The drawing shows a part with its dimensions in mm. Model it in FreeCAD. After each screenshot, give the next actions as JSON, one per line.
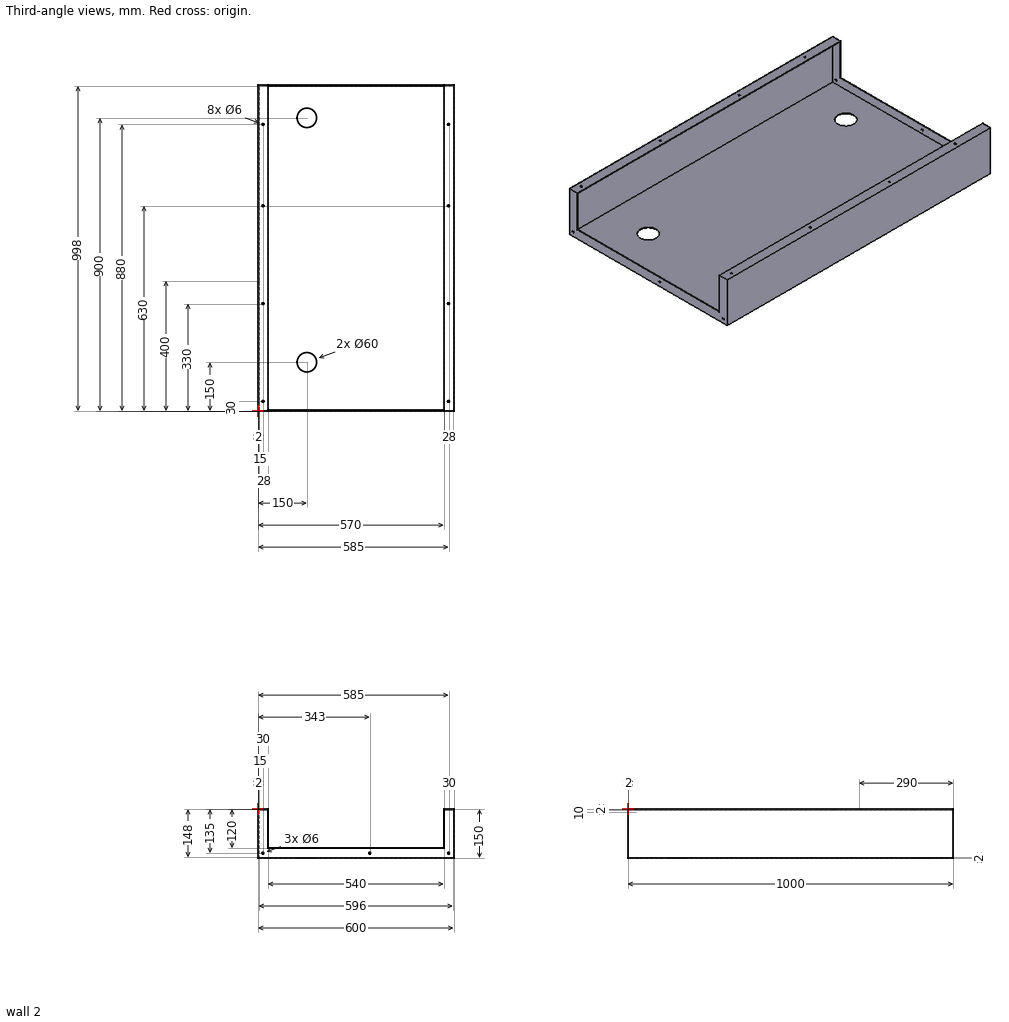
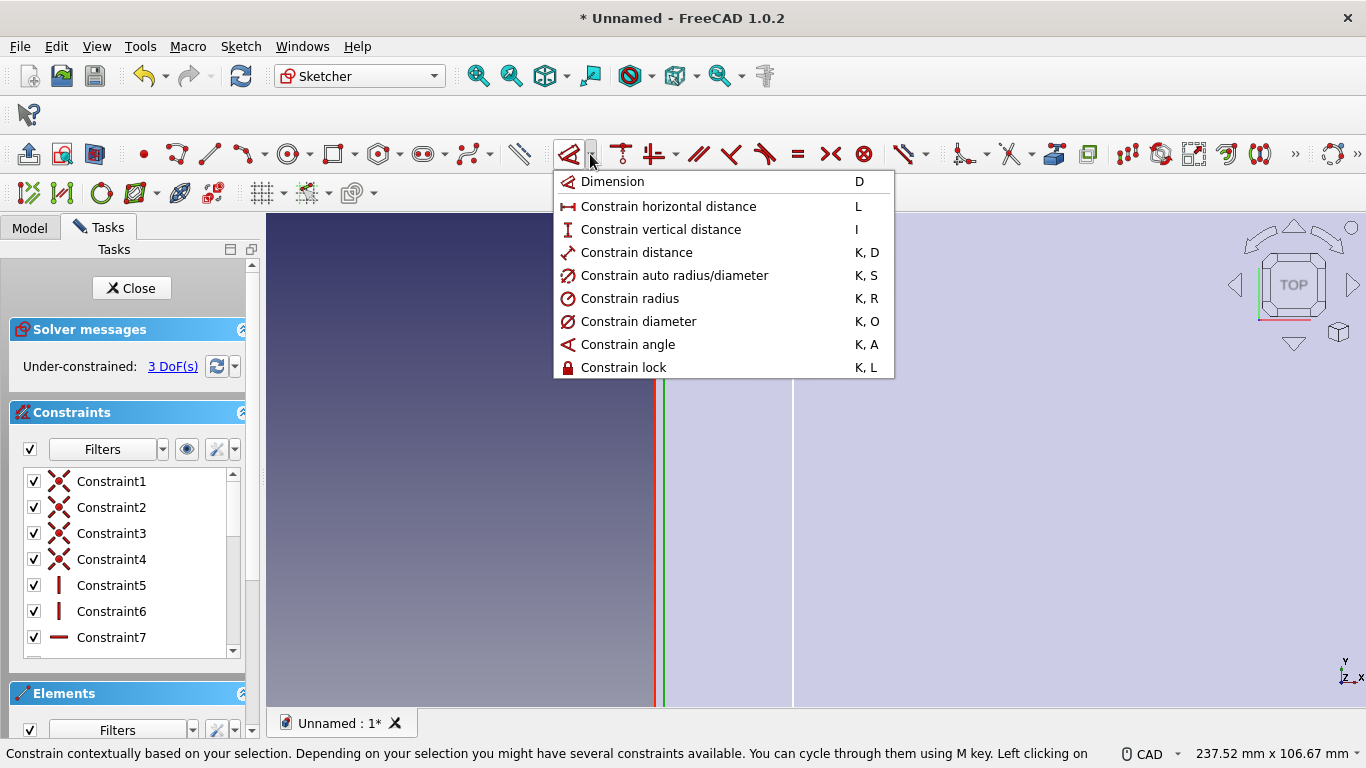
{"action": "left_click", "coordinate": [724, 230]}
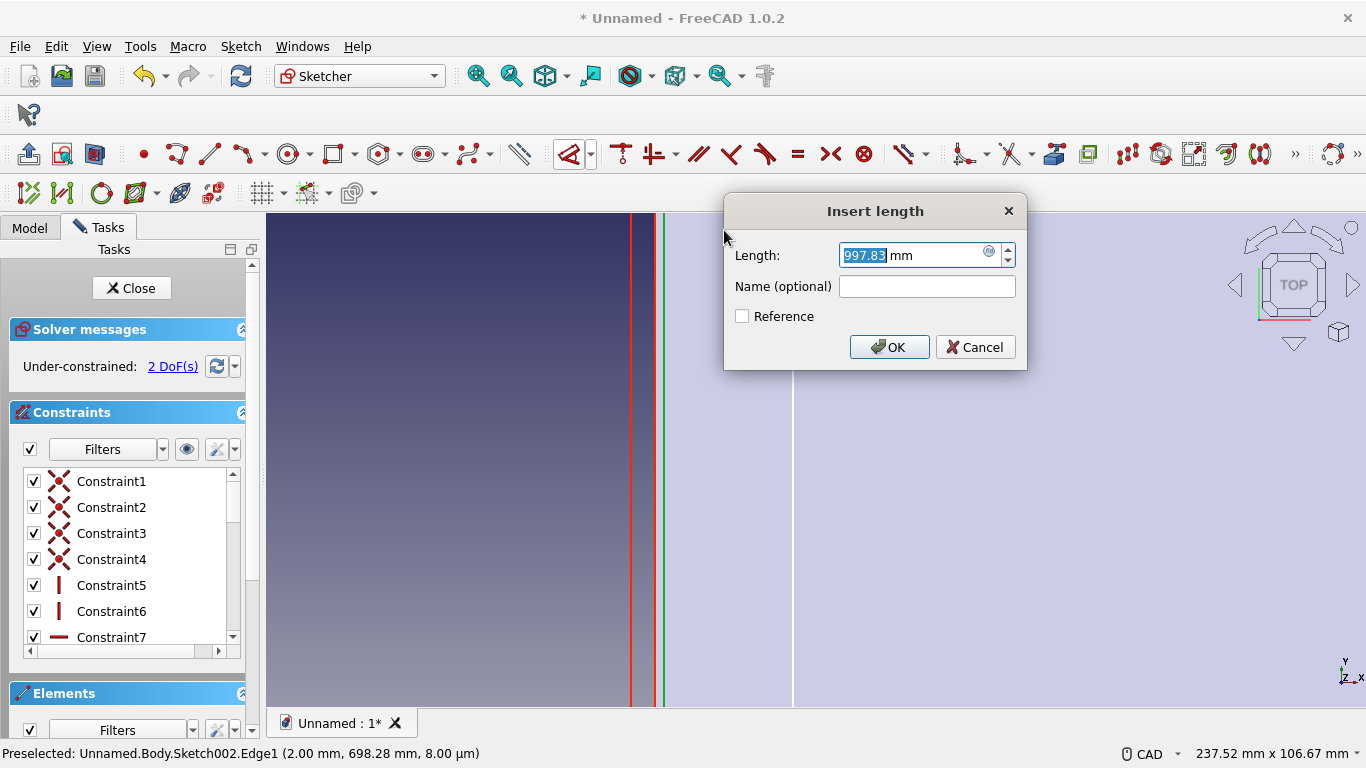
{"action": "type", "text": "998"}
{"action": "key", "text": "Return"}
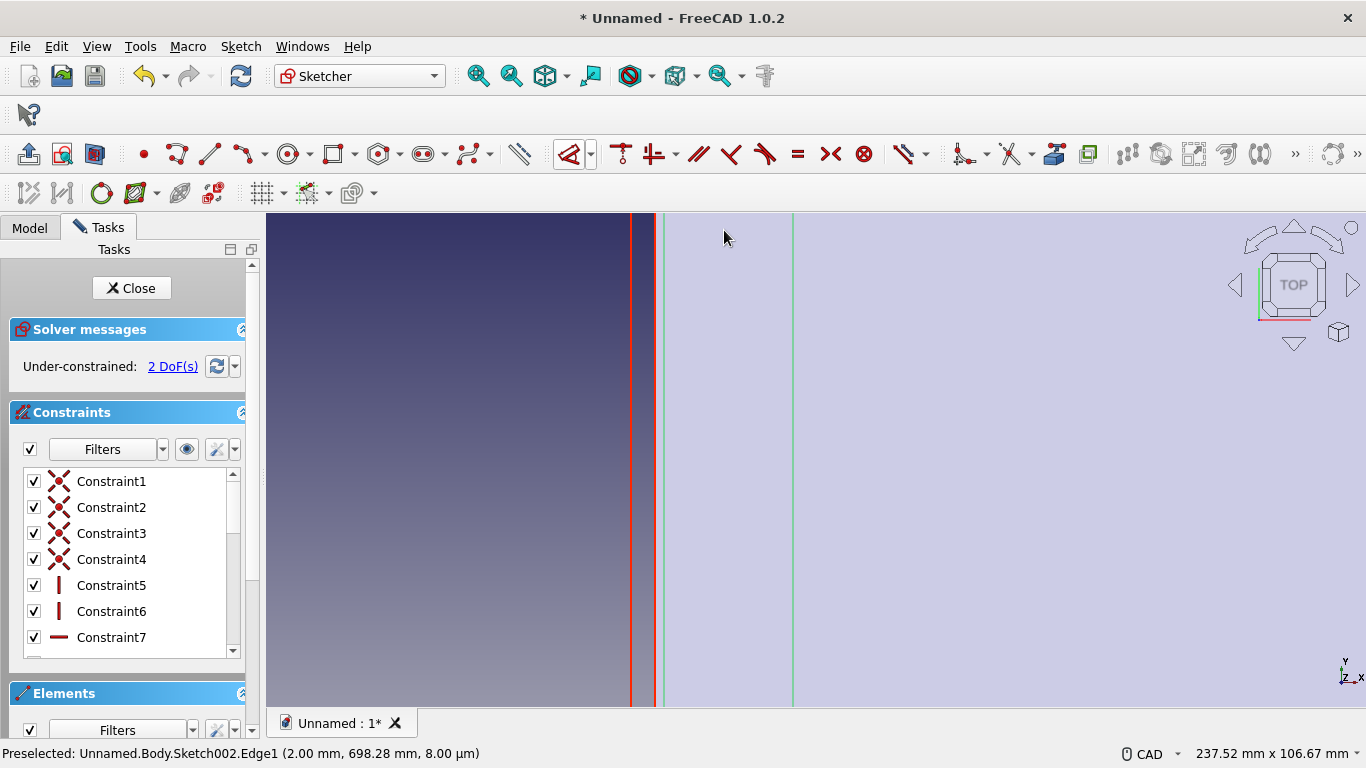
{"action": "scroll", "coordinate": [664, 405], "scroll_direction": "down", "scroll_amount": 14}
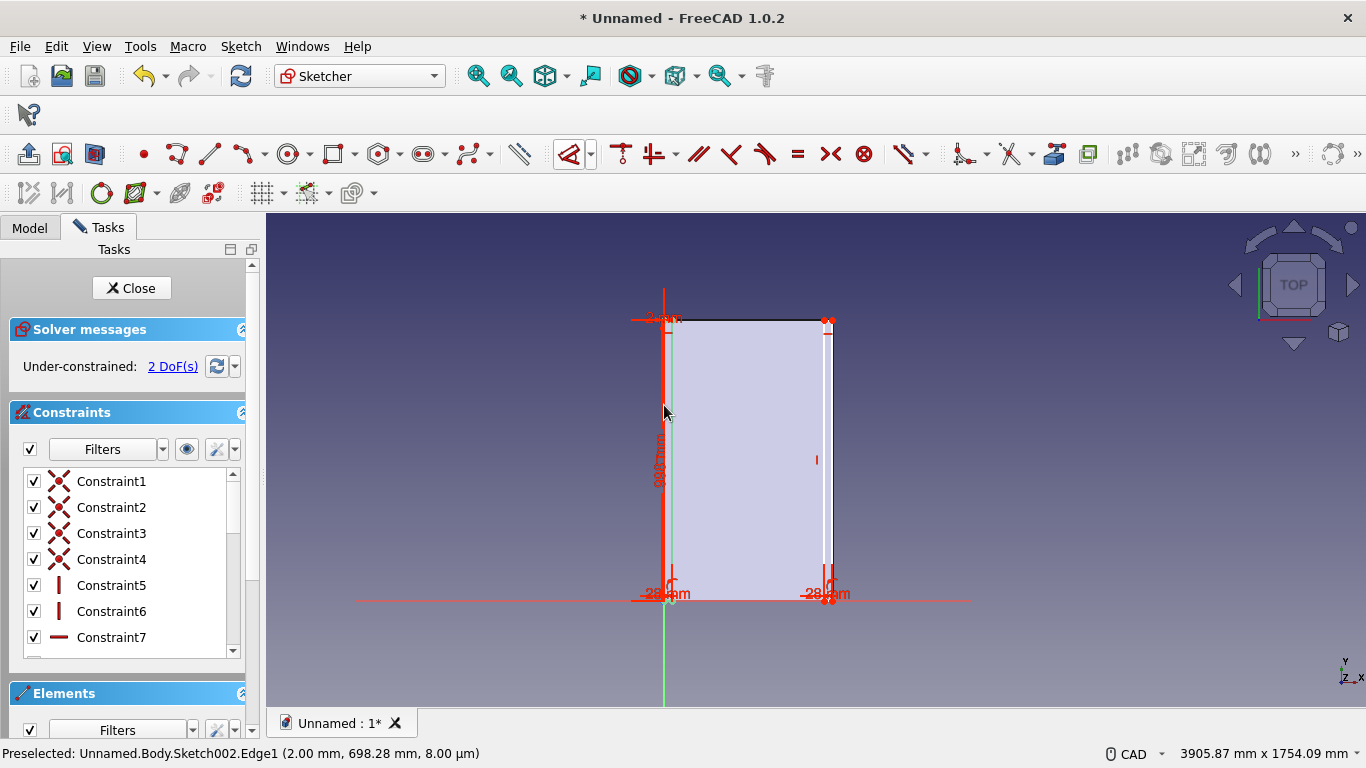
{"action": "scroll", "coordinate": [824, 405], "scroll_direction": "up", "scroll_amount": 3}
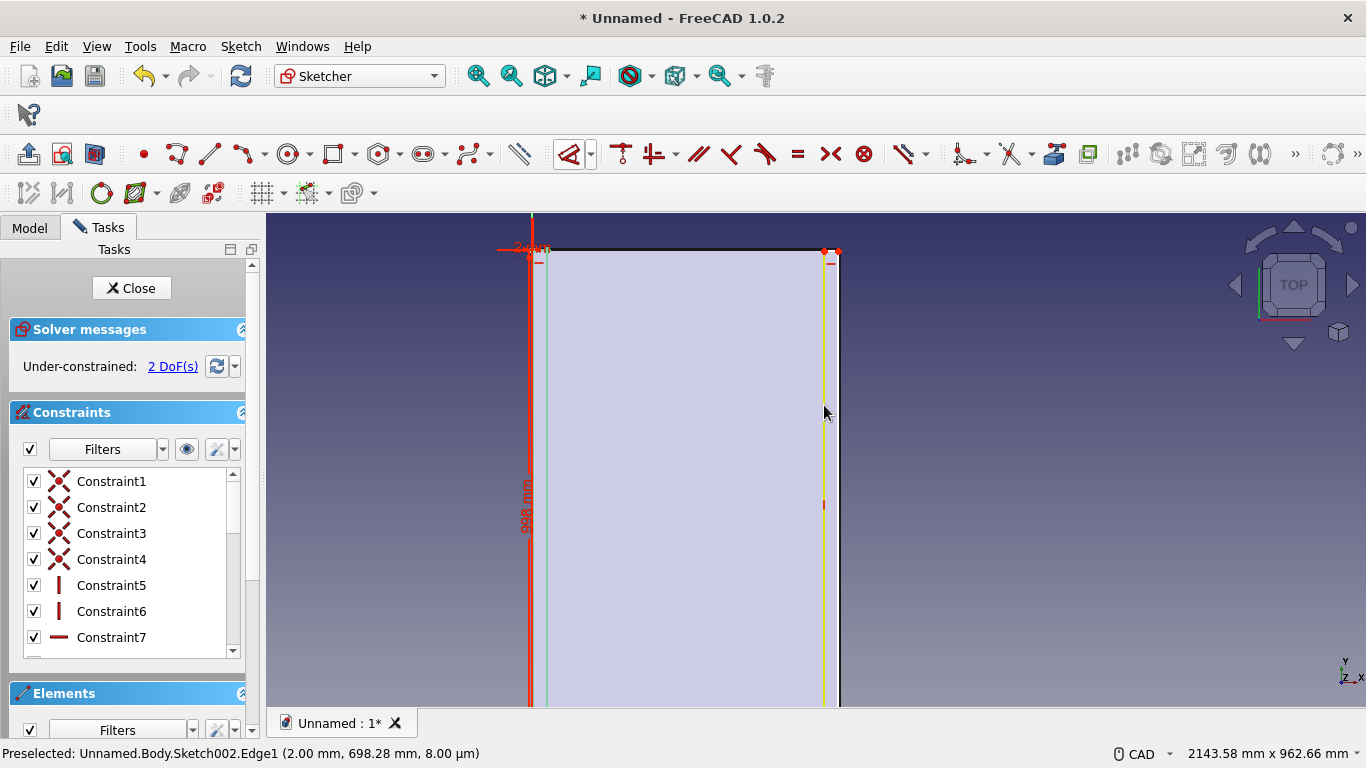
{"action": "left_click", "coordinate": [824, 405]}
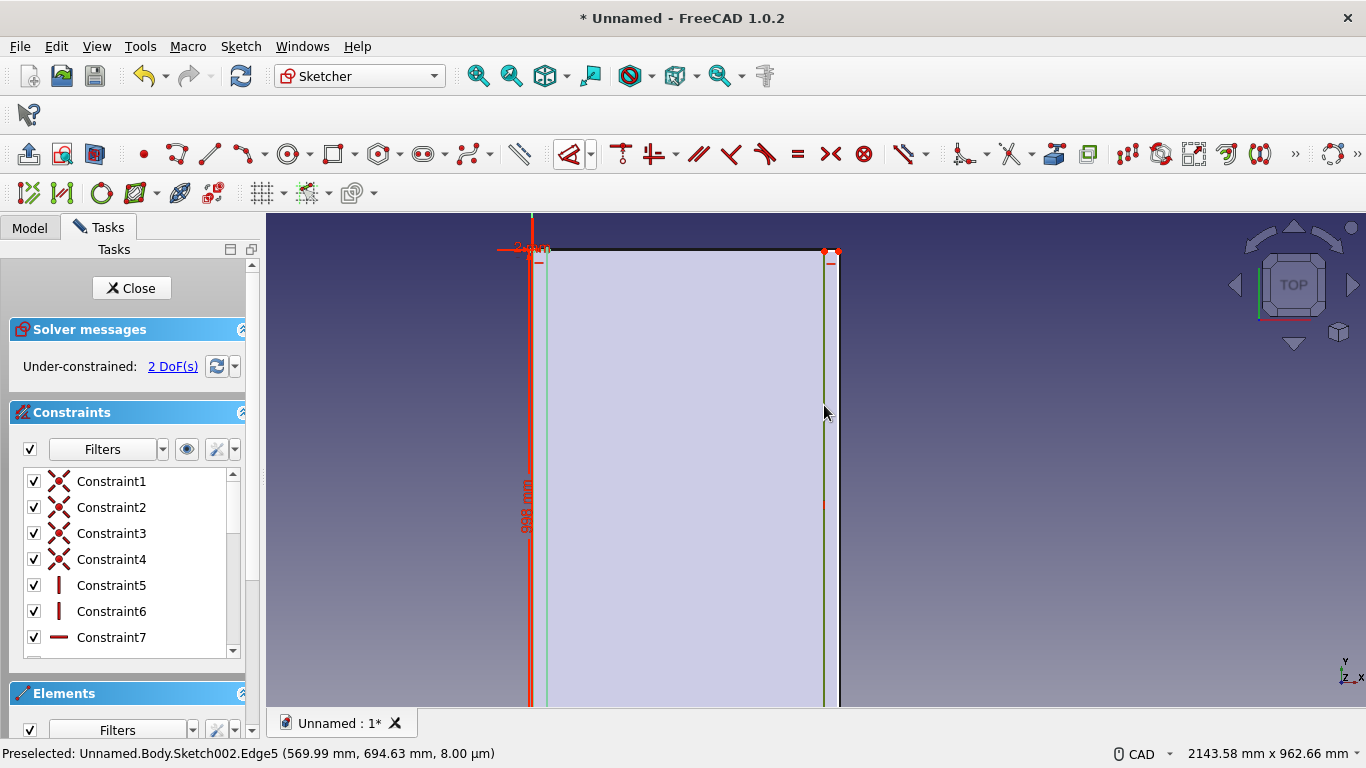
{"action": "key", "text": "i"}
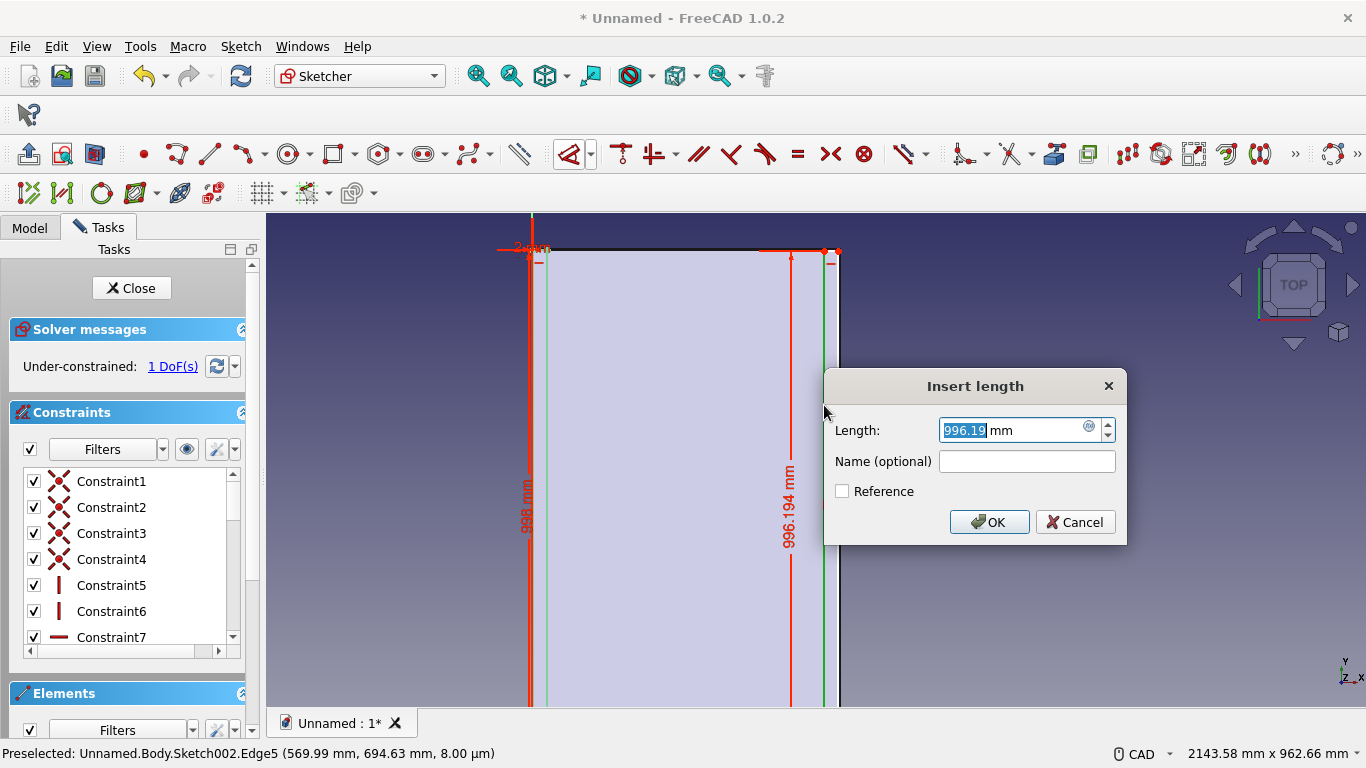
{"action": "type", "text": "998"}
{"action": "key", "text": "Return"}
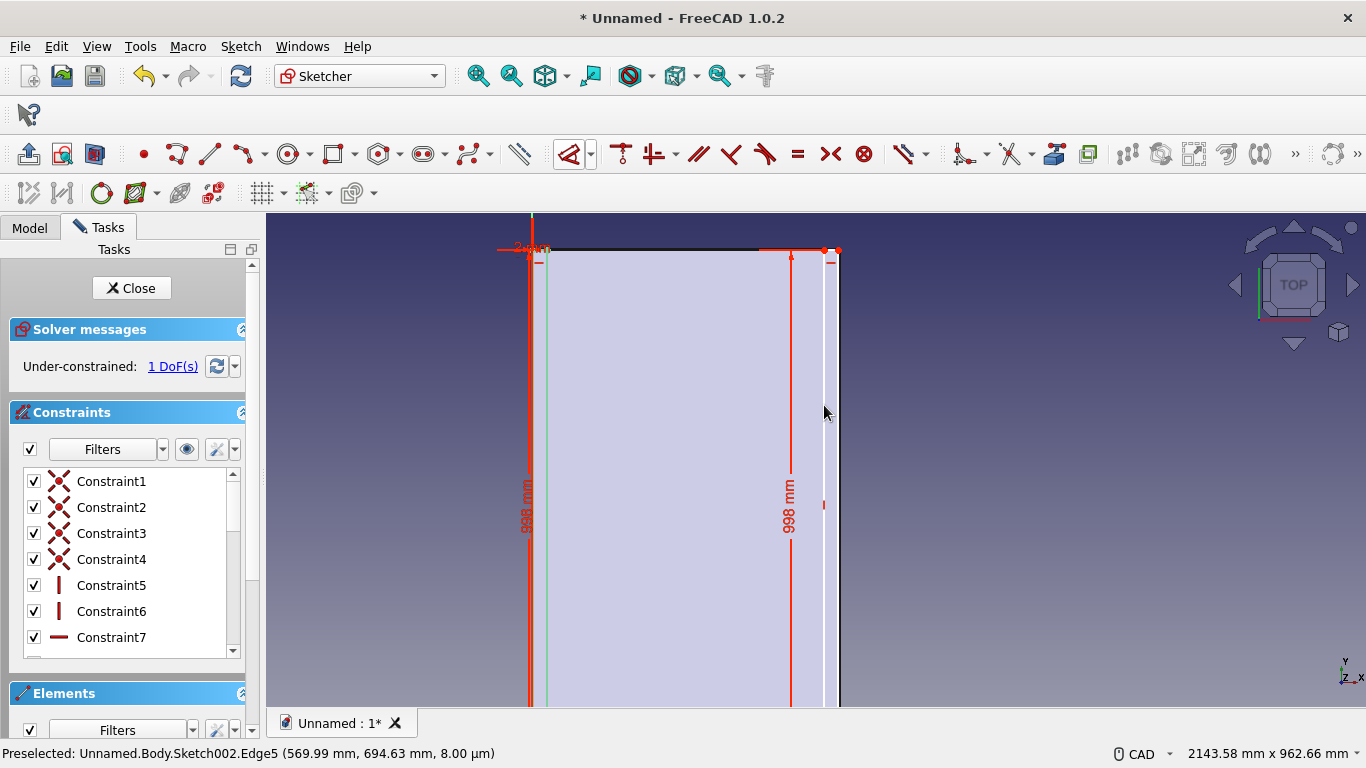
{"action": "left_click", "coordinate": [824, 250]}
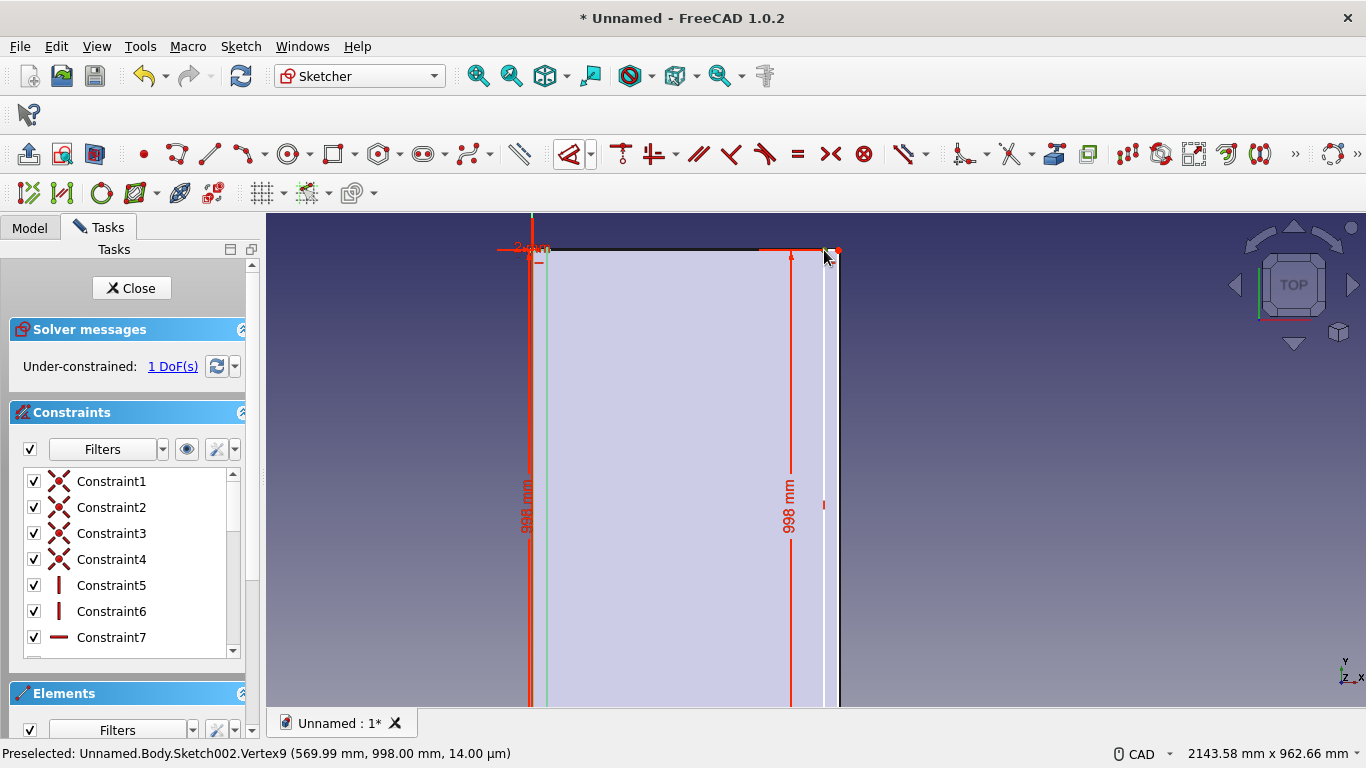
{"action": "key", "text": "l"}